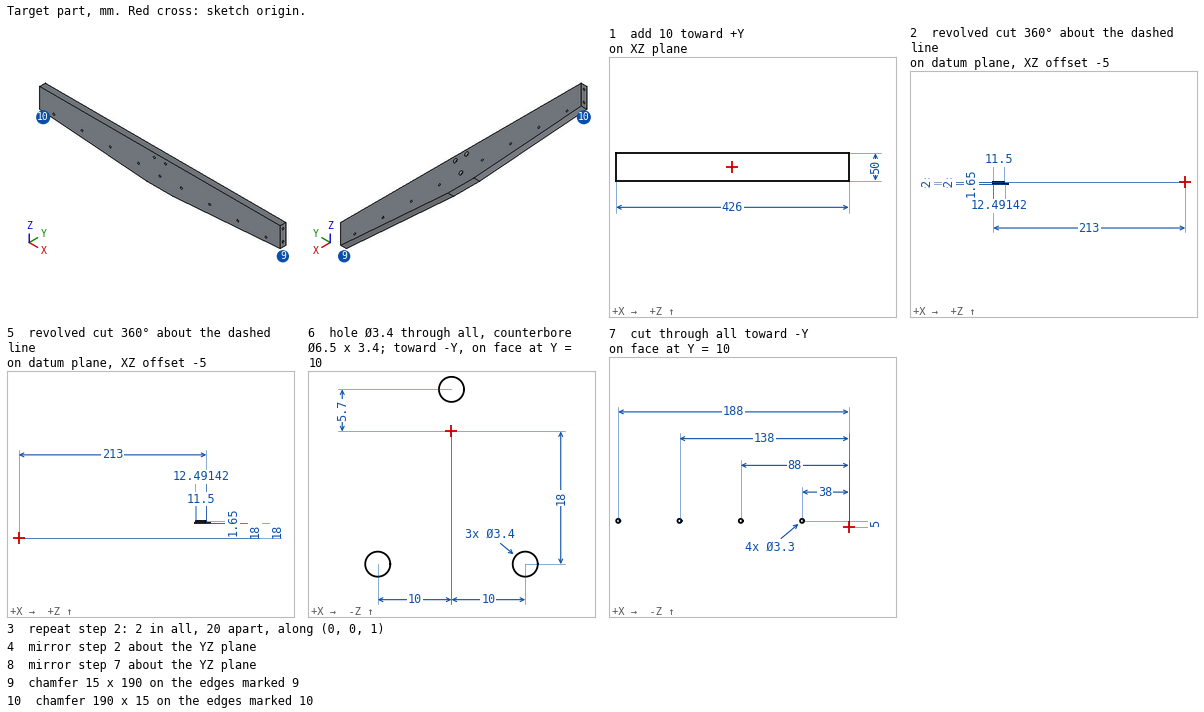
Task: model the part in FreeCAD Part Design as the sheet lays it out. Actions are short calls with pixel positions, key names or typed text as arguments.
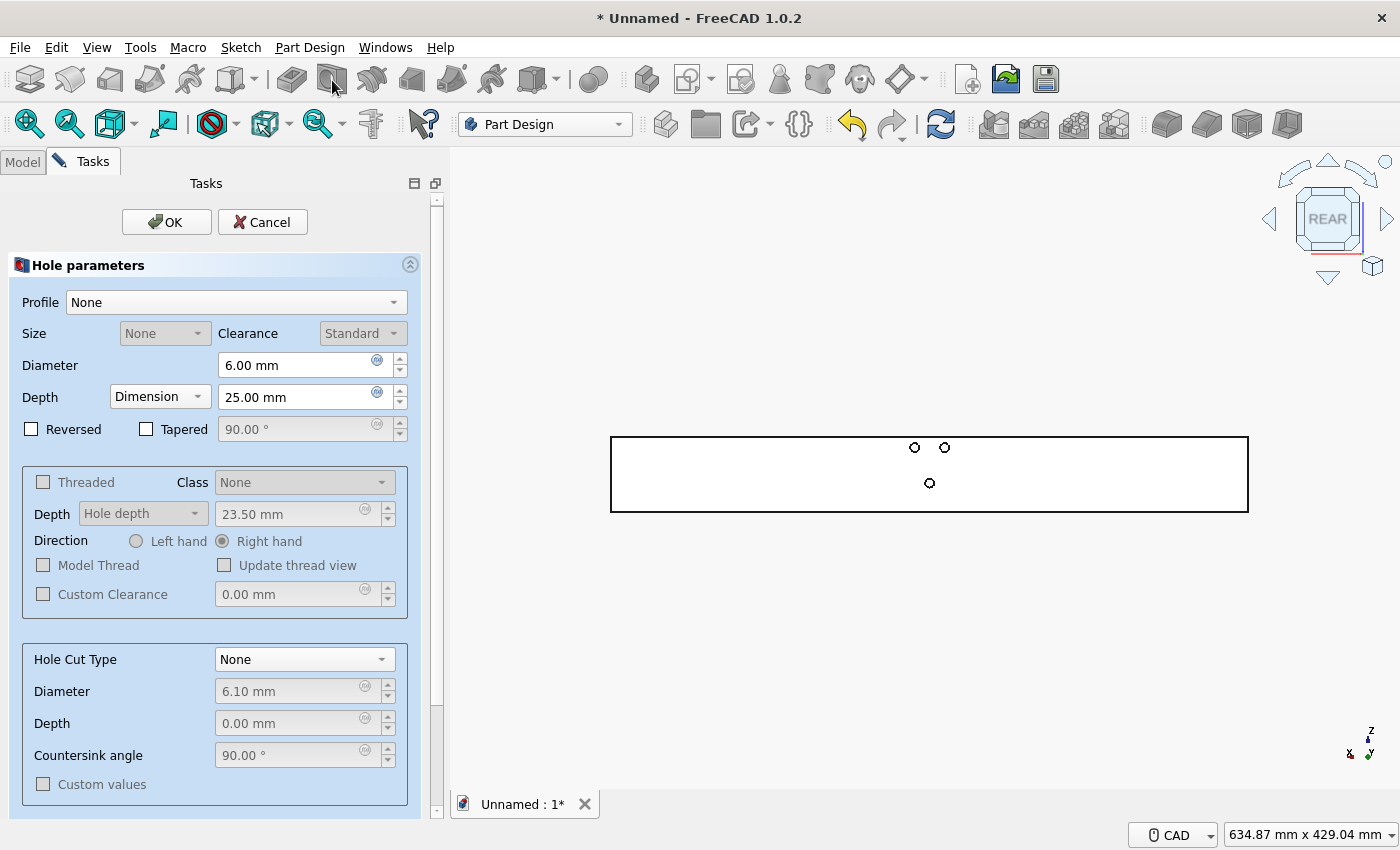
triple_click(305, 365)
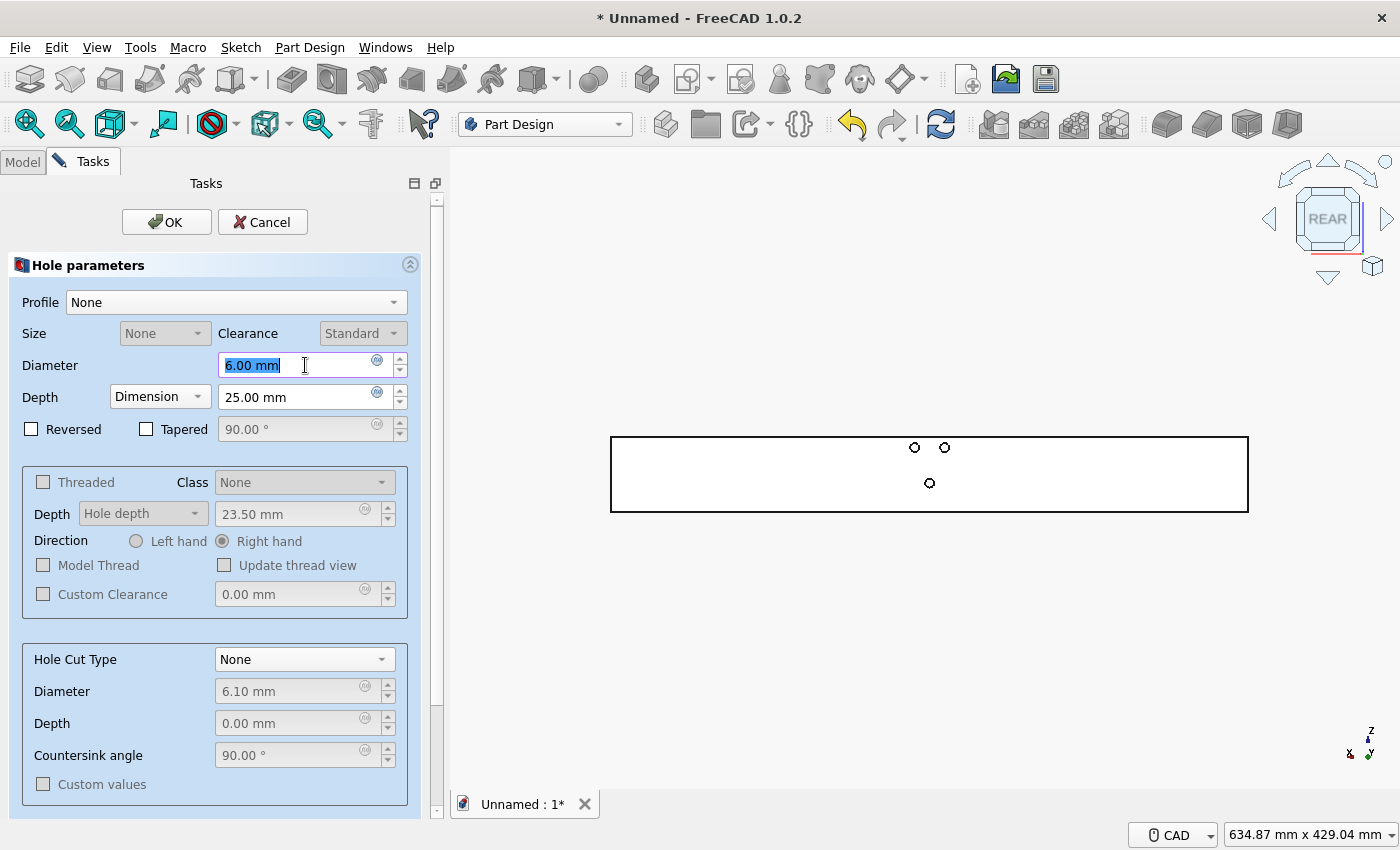
text(3.4)
key(Tab)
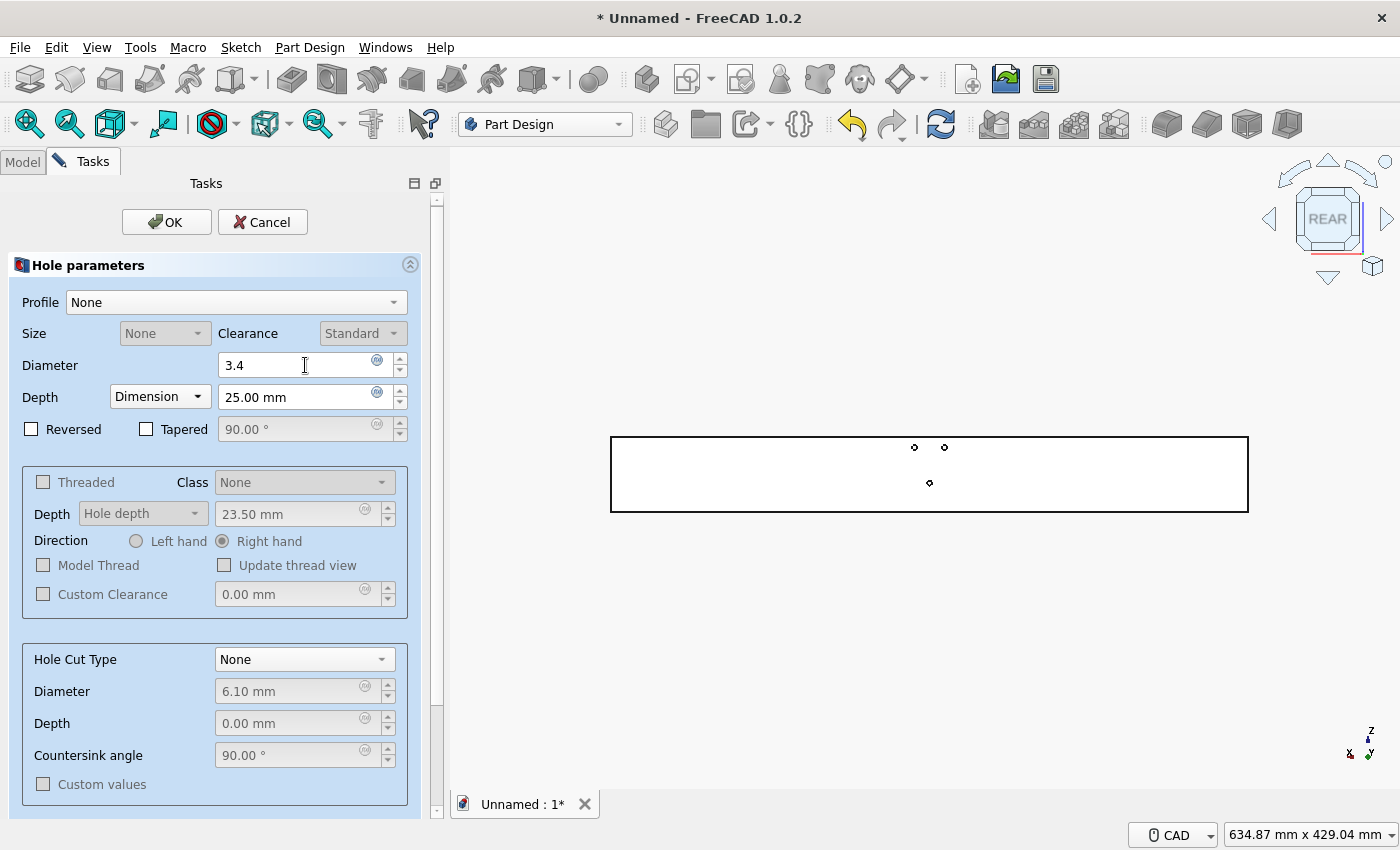
click(161, 396)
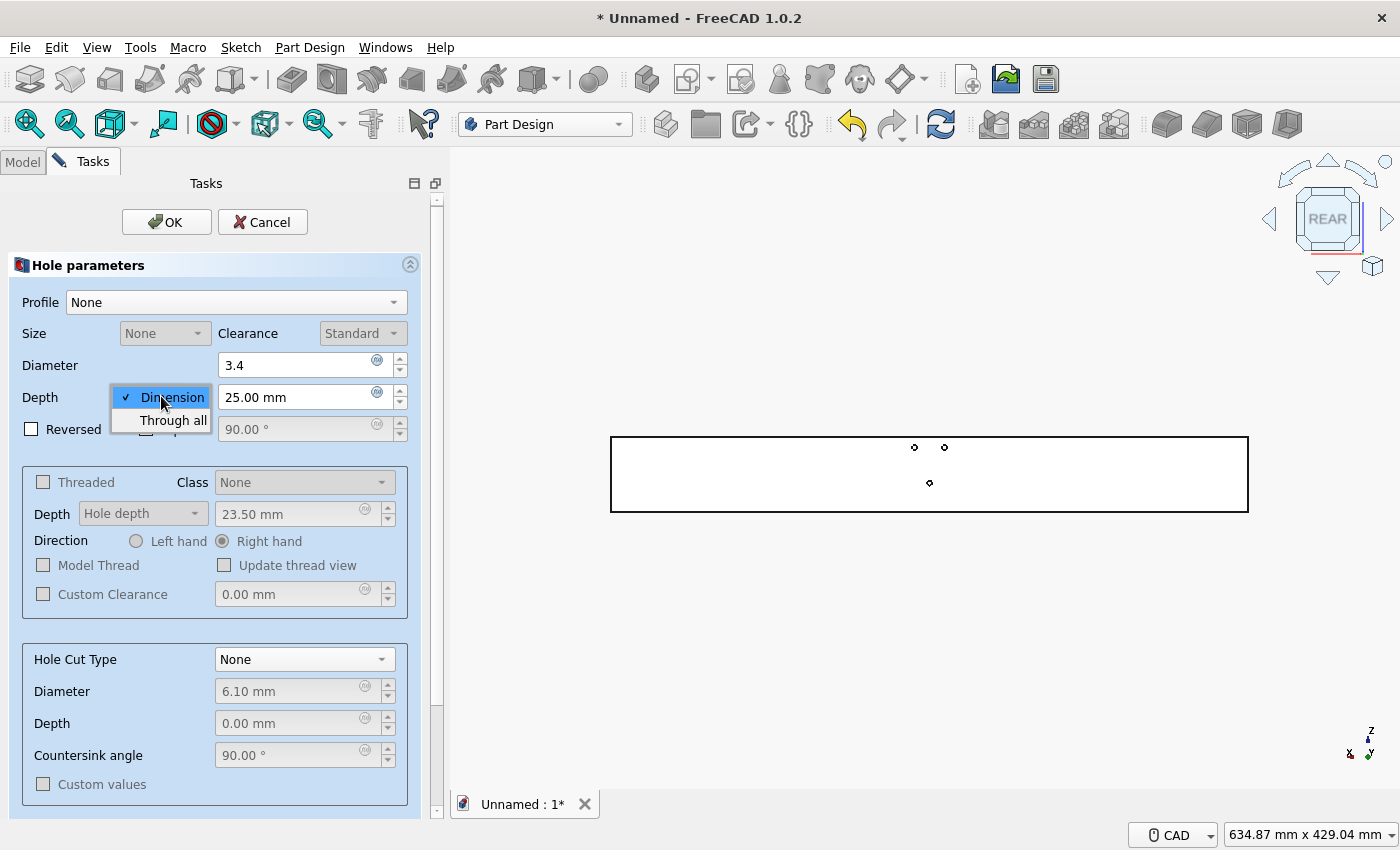
click(160, 420)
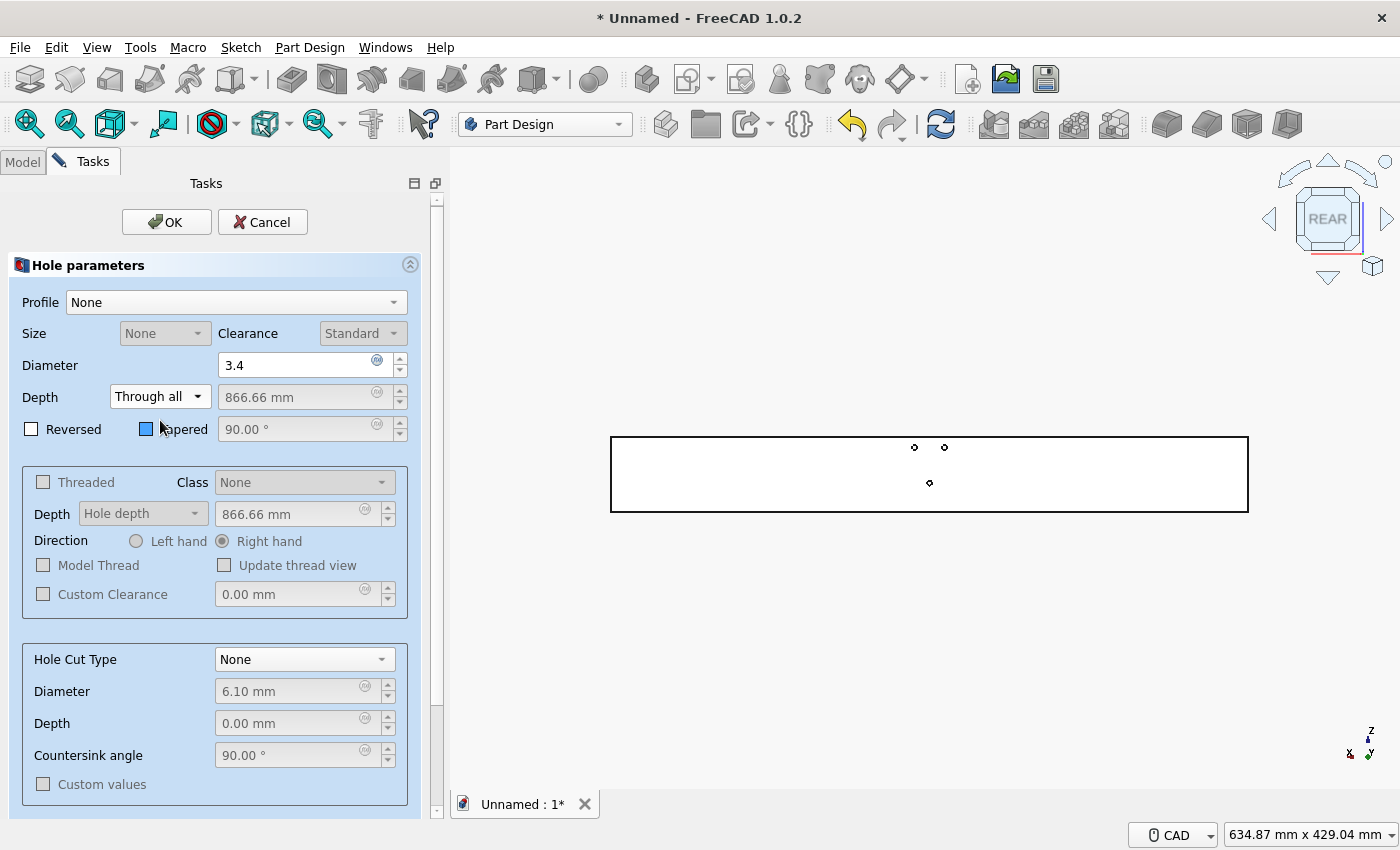
click(306, 660)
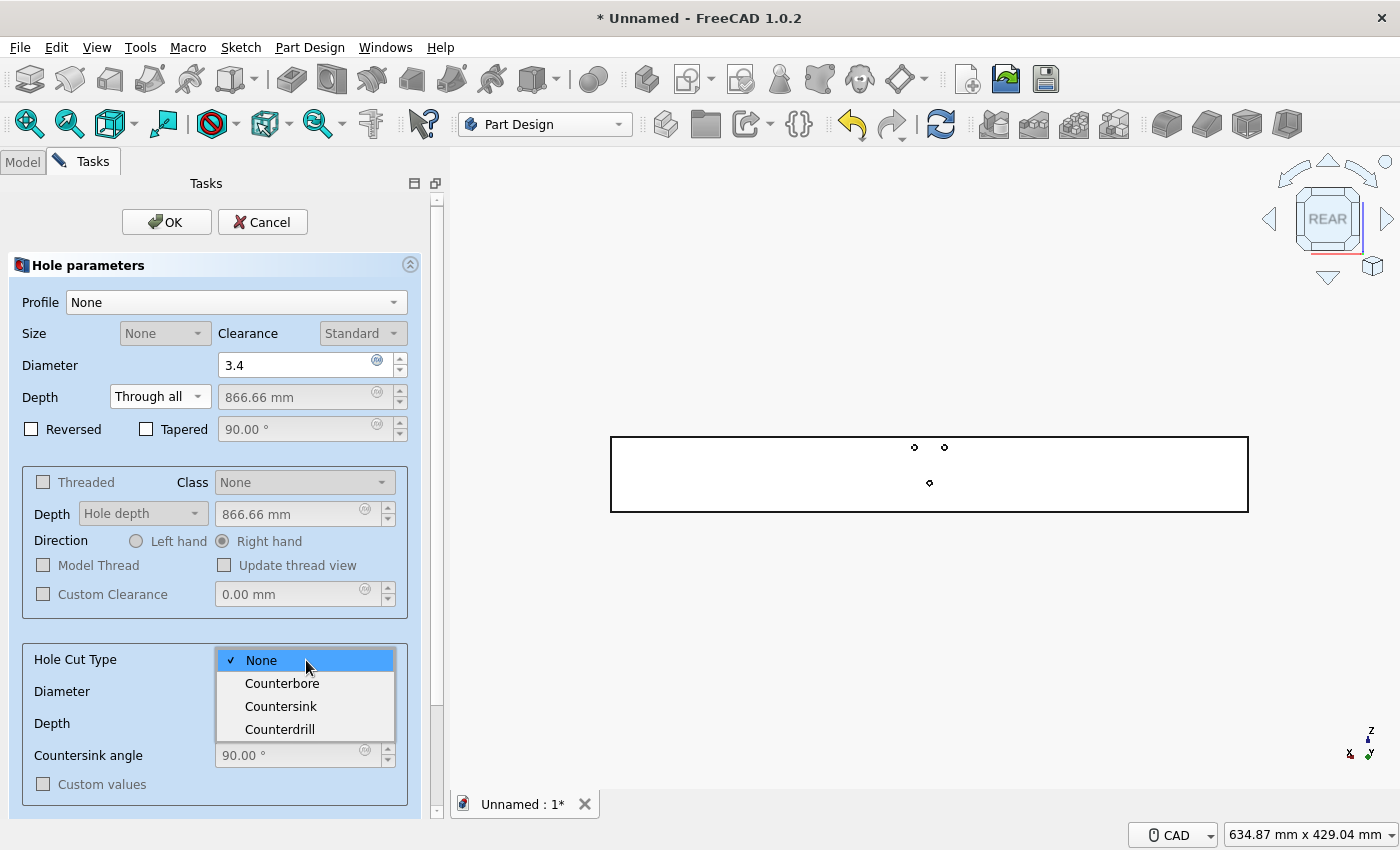
click(304, 684)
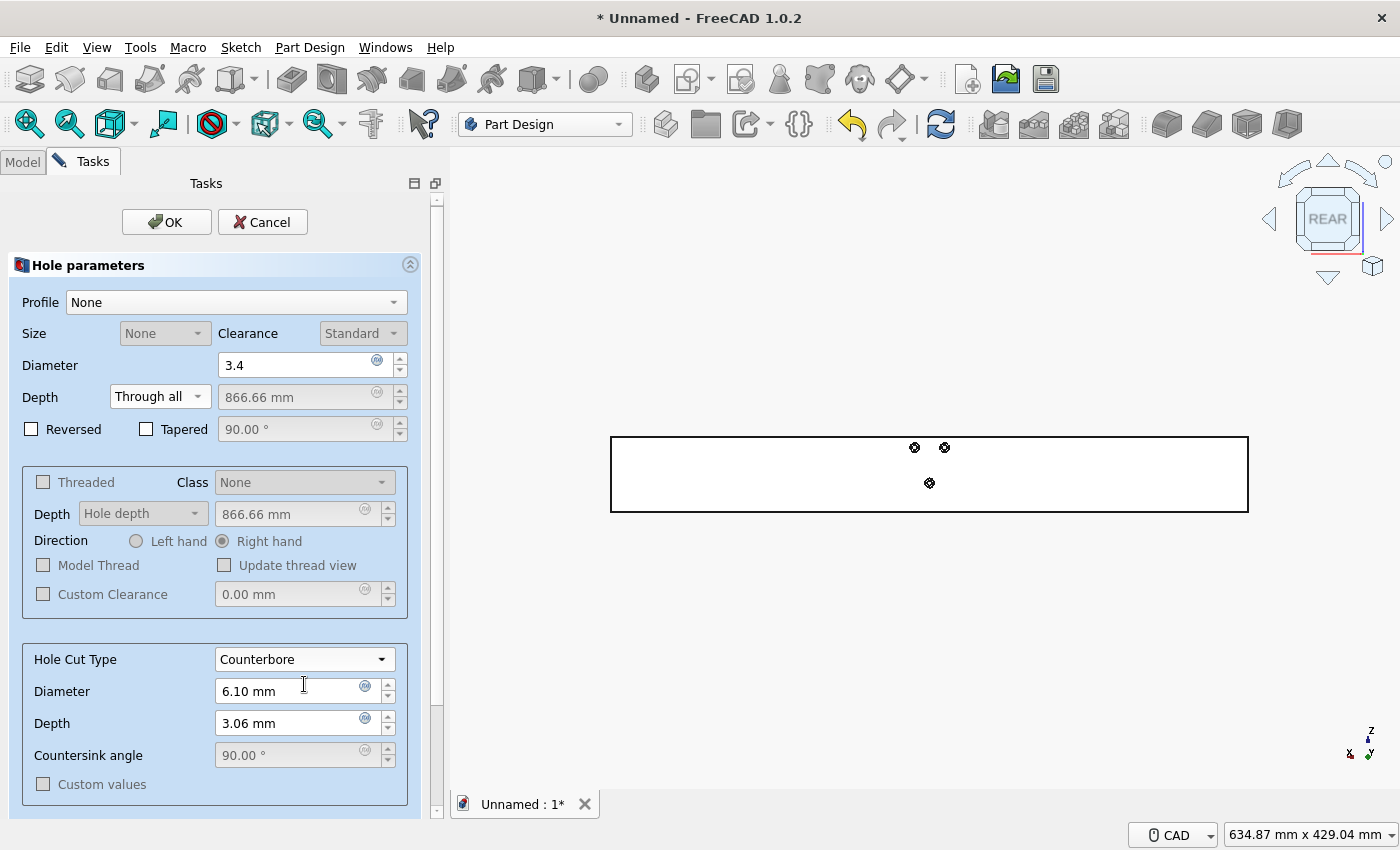
triple_click(298, 691)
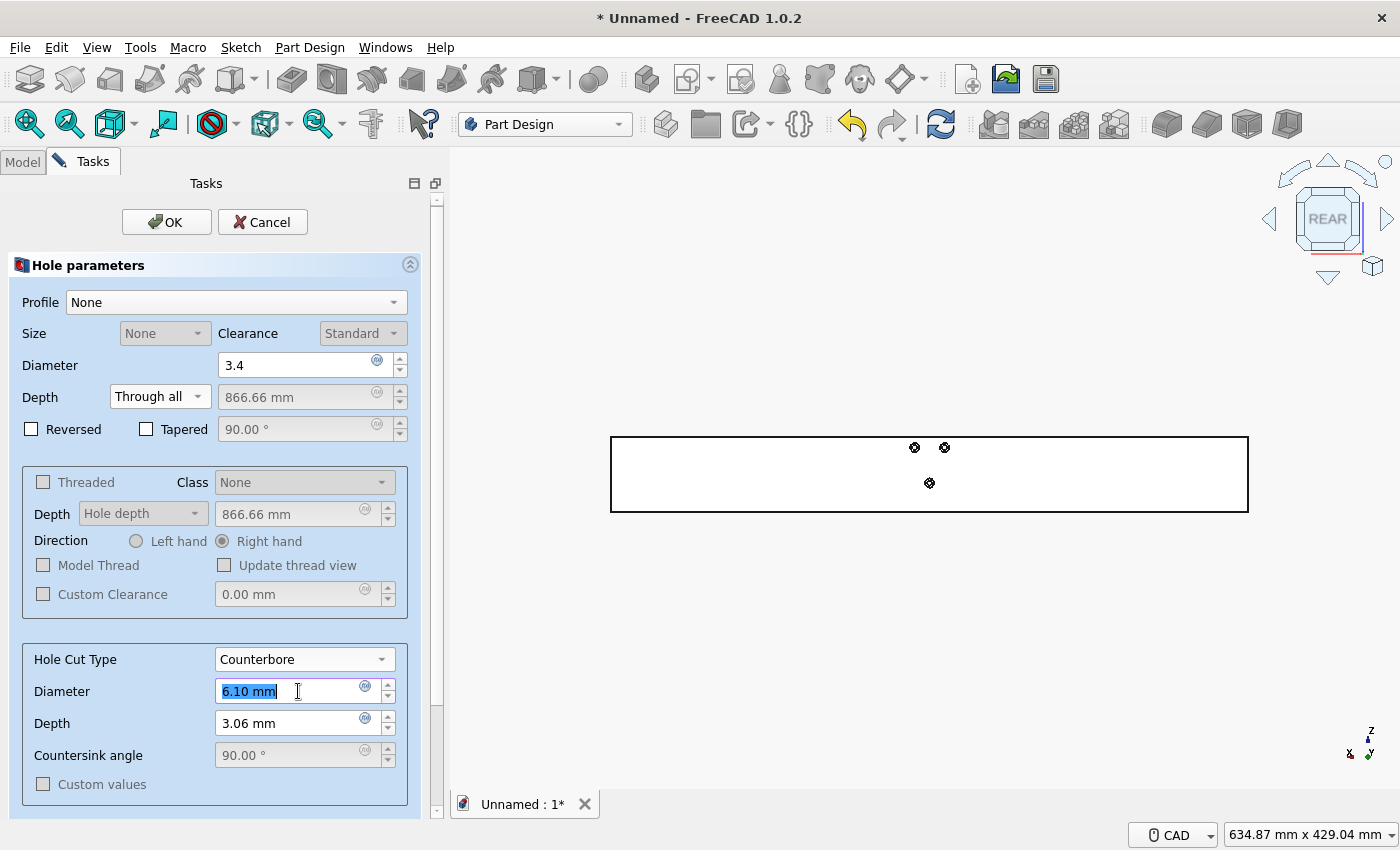
text(6.5)
key(Tab)